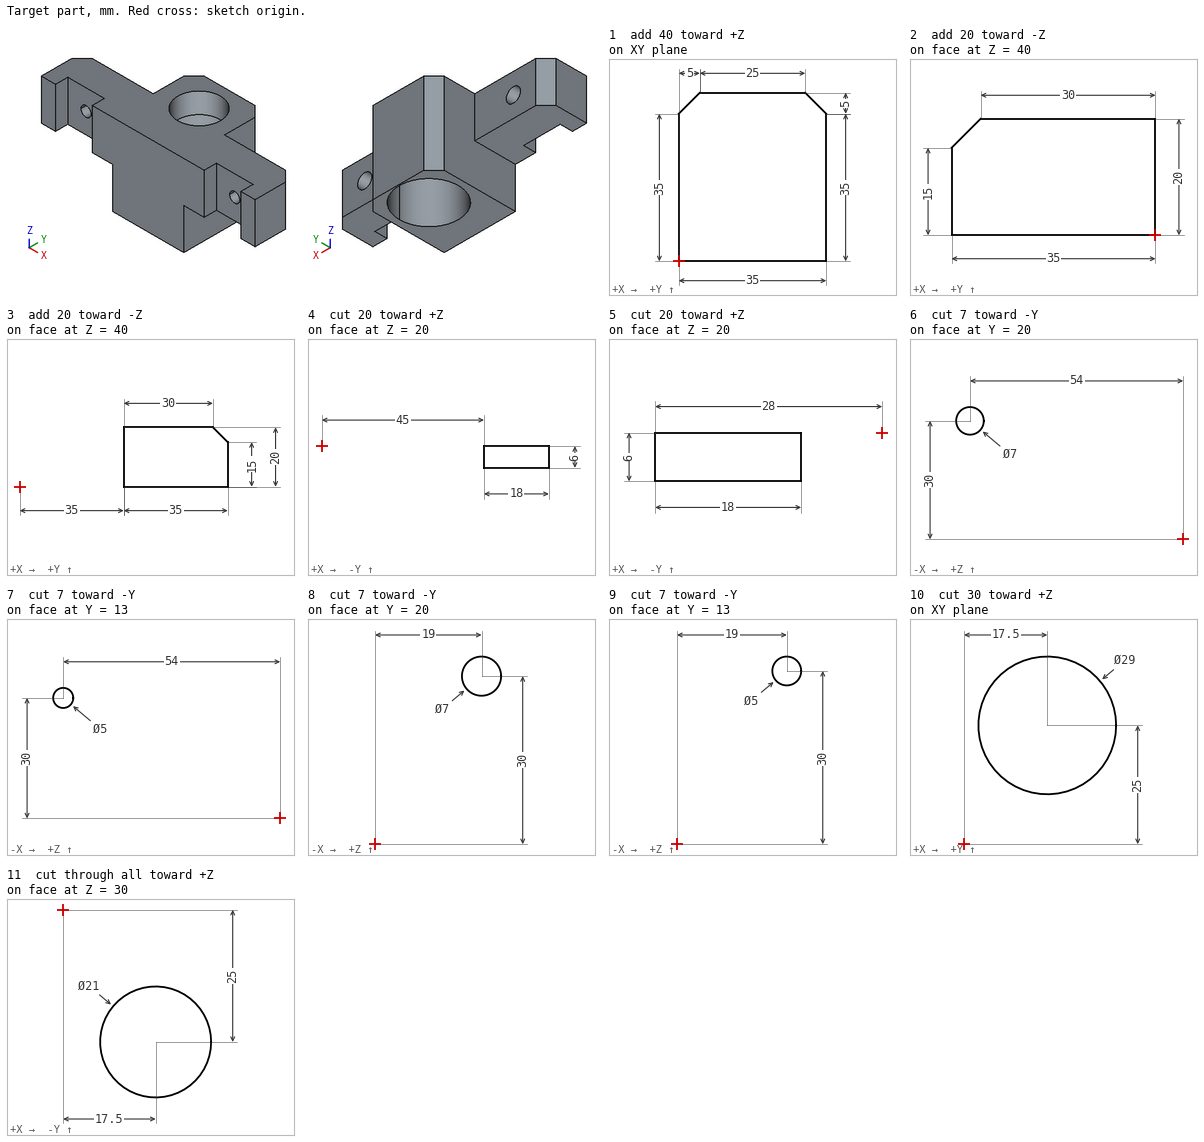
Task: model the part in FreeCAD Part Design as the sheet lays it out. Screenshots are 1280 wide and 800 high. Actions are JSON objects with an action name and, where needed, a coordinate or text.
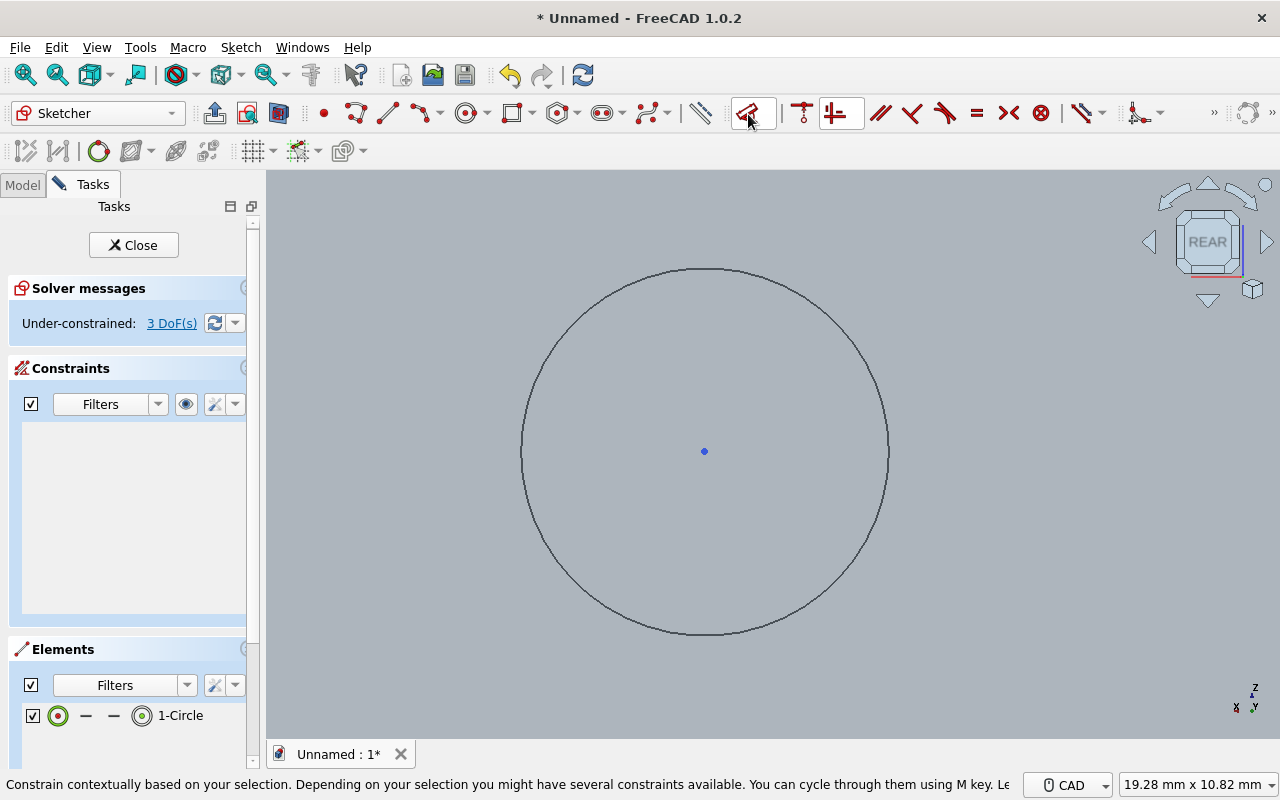
{"action": "left_click", "coordinate": [835, 322]}
{"action": "left_click", "coordinate": [858, 299]}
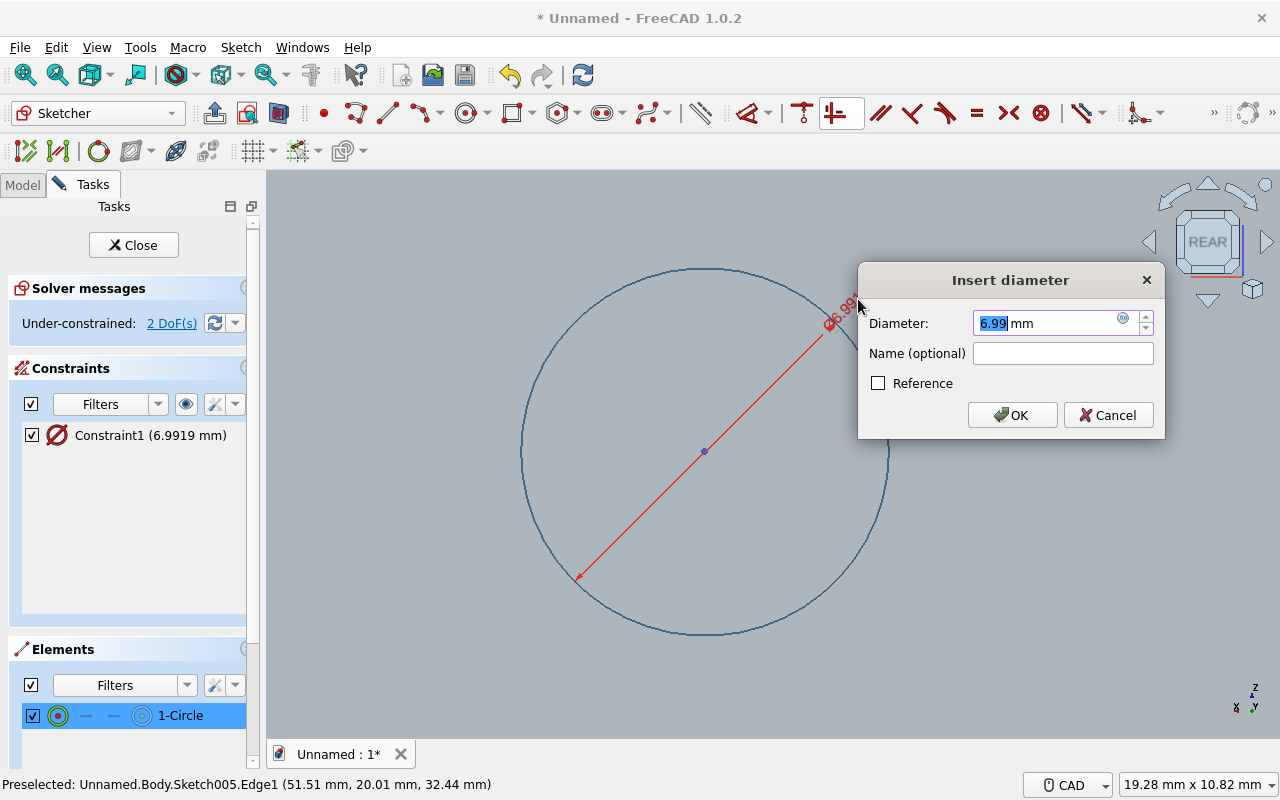
{"action": "type", "text": "7"}
{"action": "key", "text": "Return"}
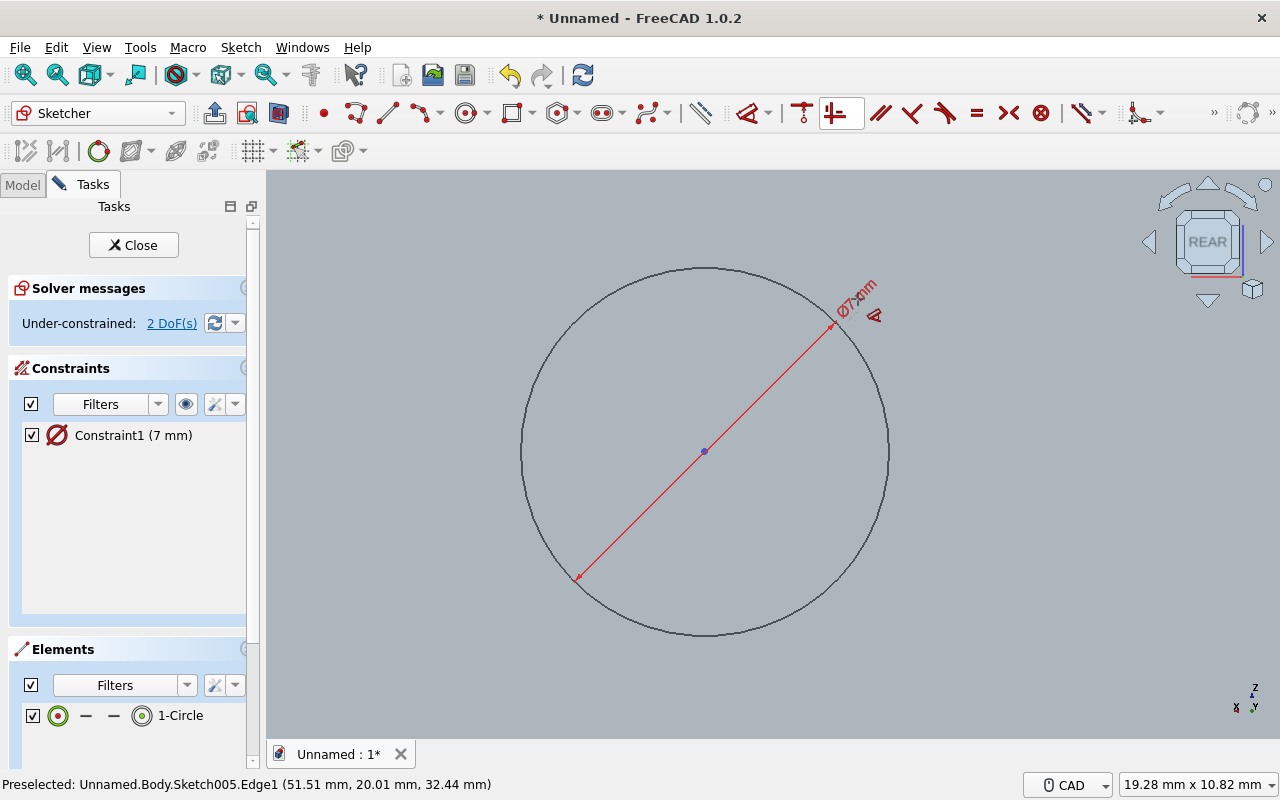
{"action": "left_click", "coordinate": [705, 452]}
{"action": "left_click", "coordinate": [910, 418]}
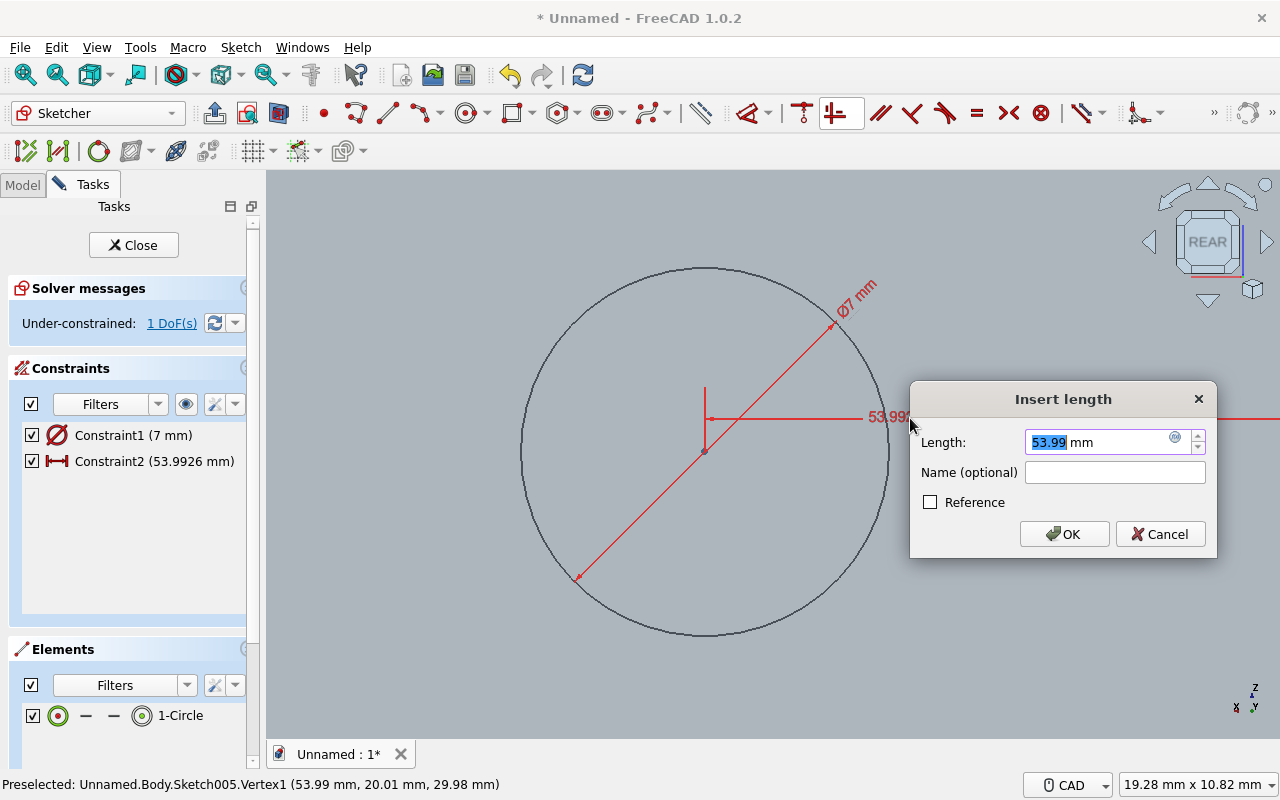
{"action": "type", "text": "54"}
{"action": "key", "text": "Return"}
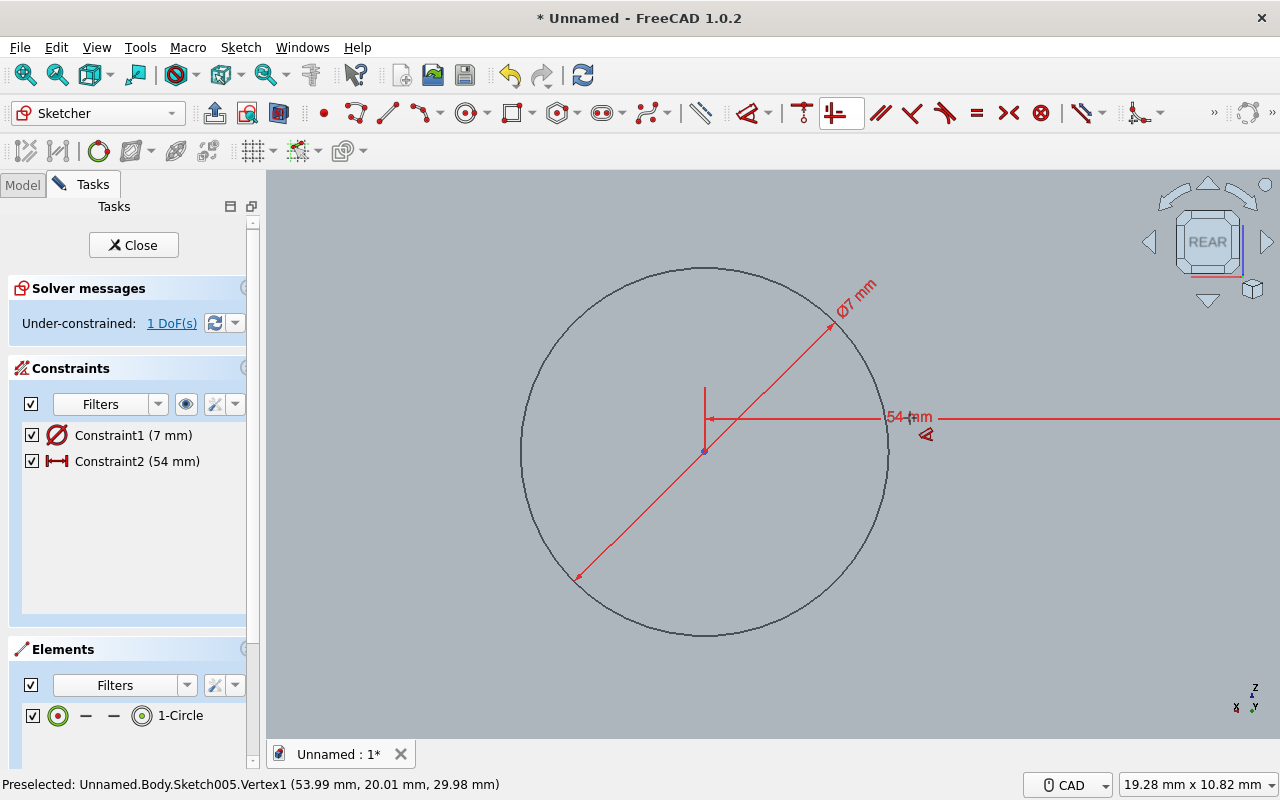
{"action": "left_click", "coordinate": [705, 452]}
{"action": "left_click", "coordinate": [671, 581]}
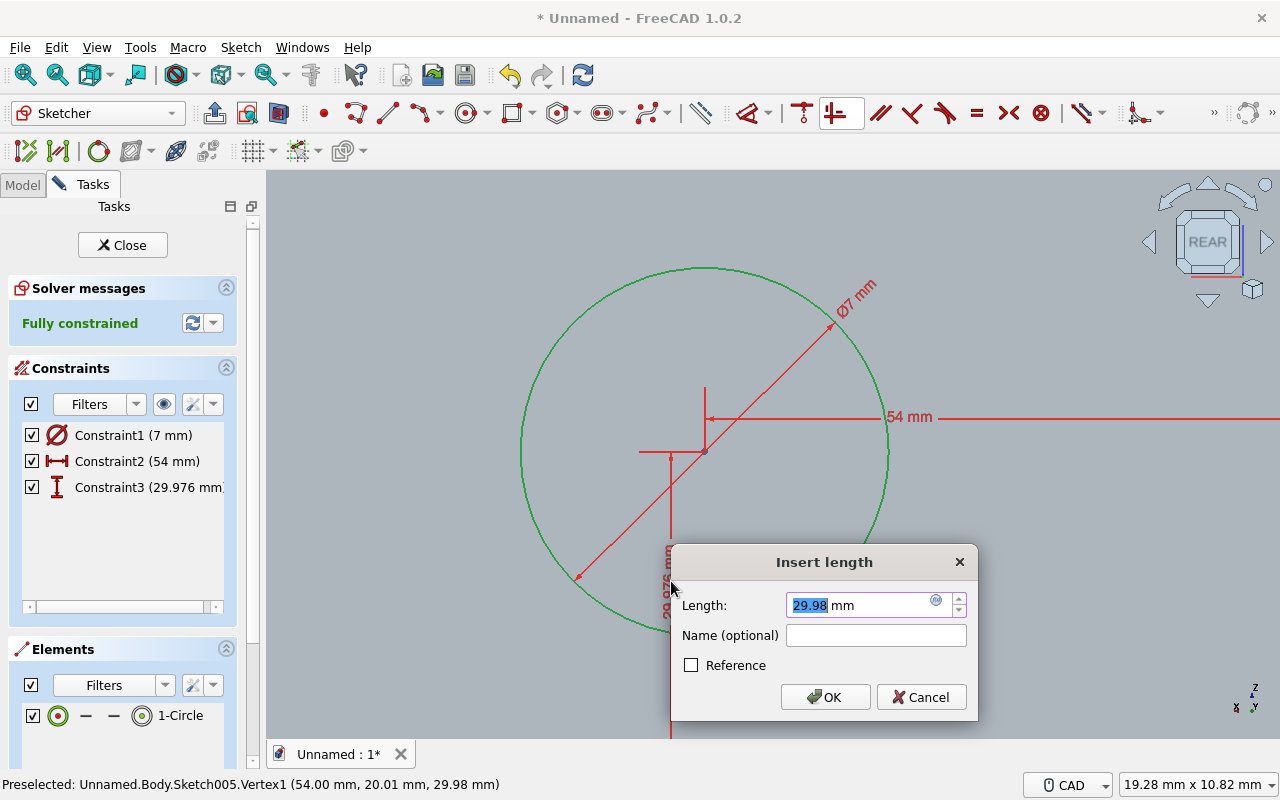
{"action": "type", "text": "30"}
{"action": "key", "text": "Return"}
{"action": "key", "text": "Escape"}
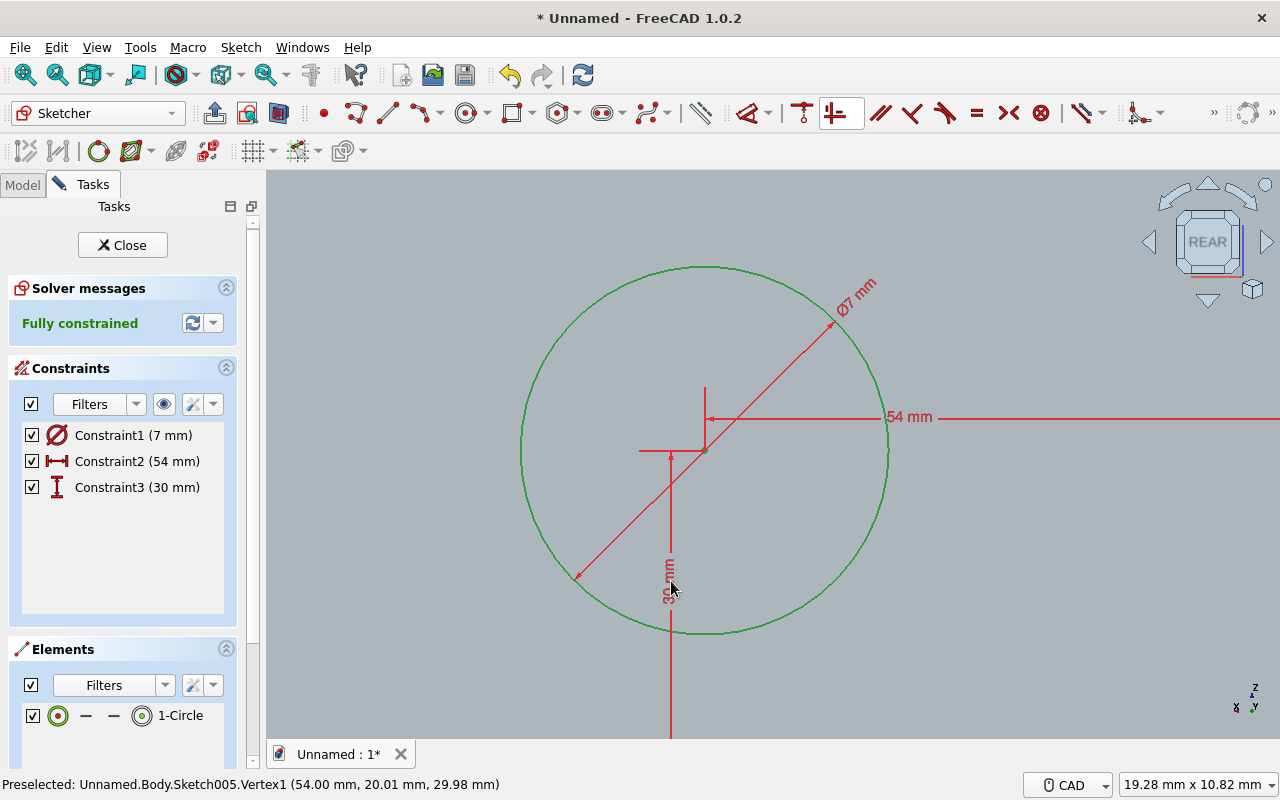
{"action": "left_click", "coordinate": [123, 245]}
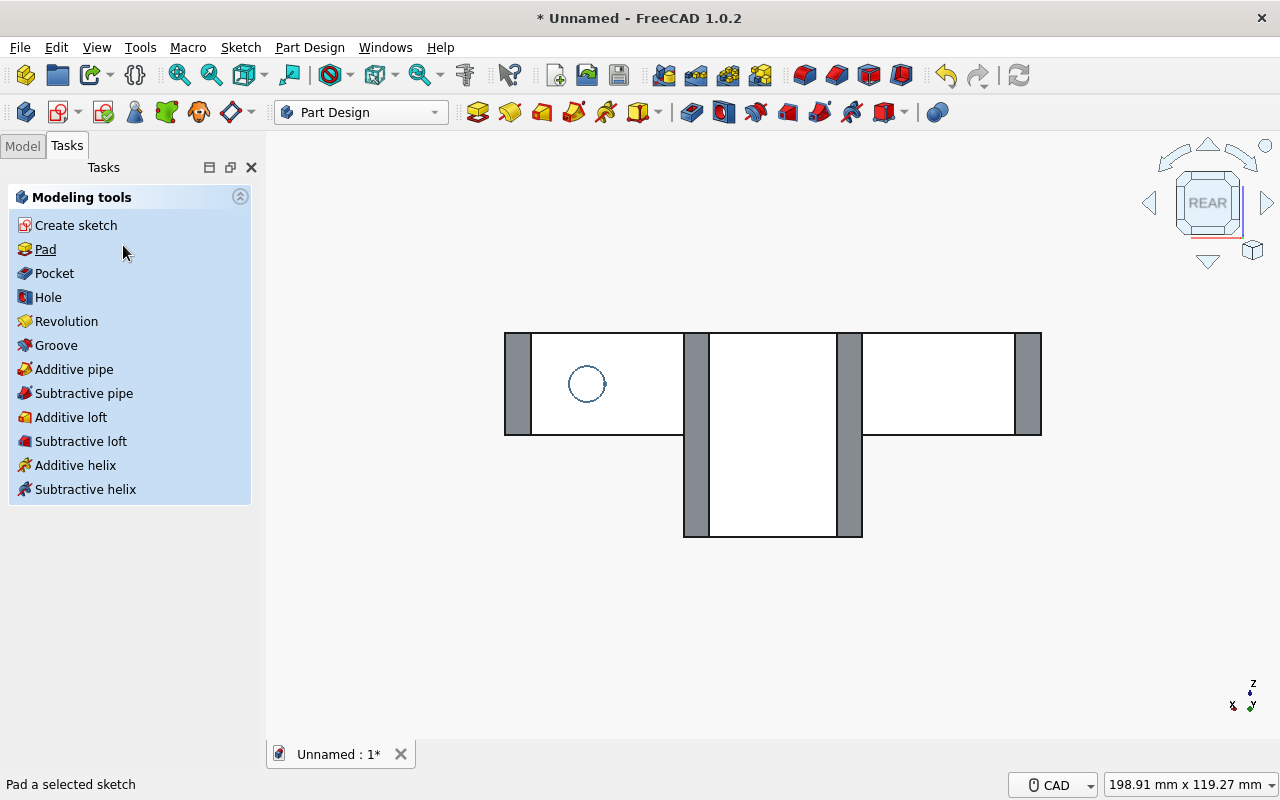
{"action": "left_click", "coordinate": [692, 112]}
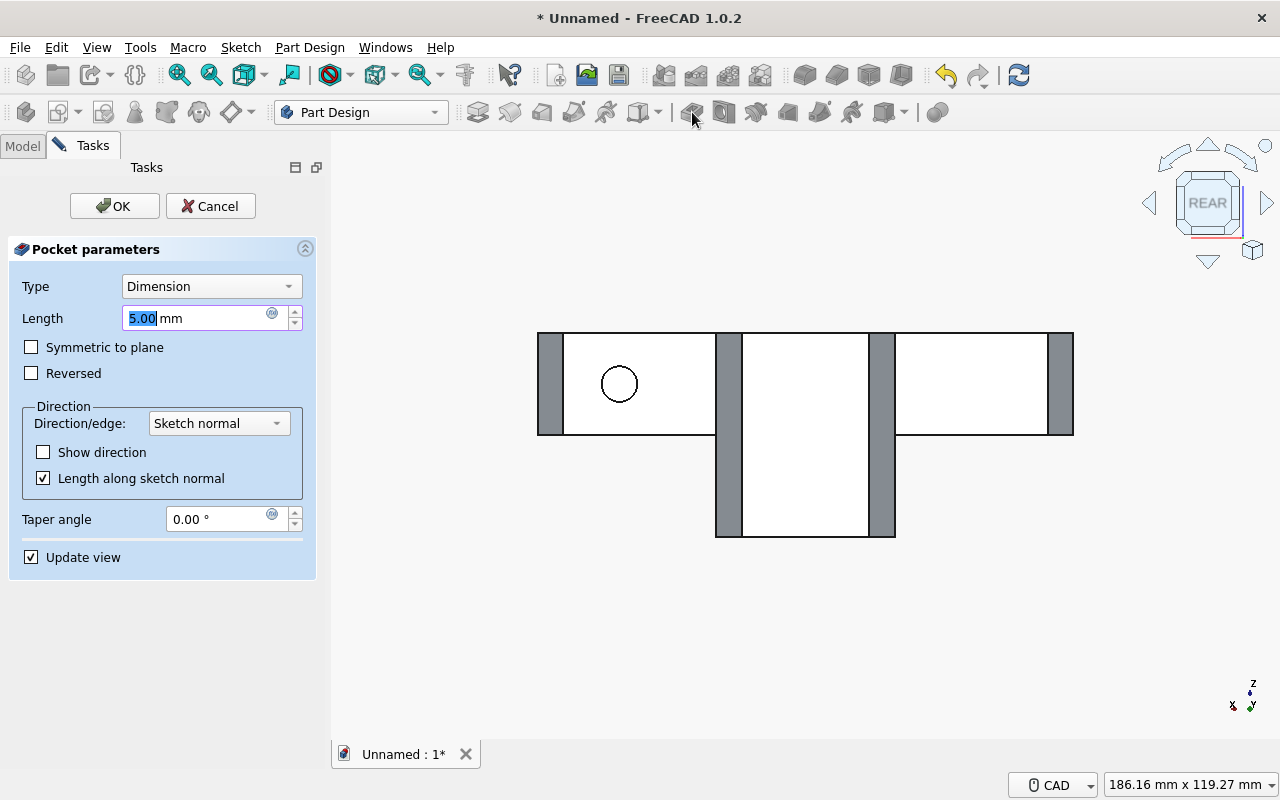
{"action": "type", "text": "7"}
{"action": "key", "text": "Tab"}